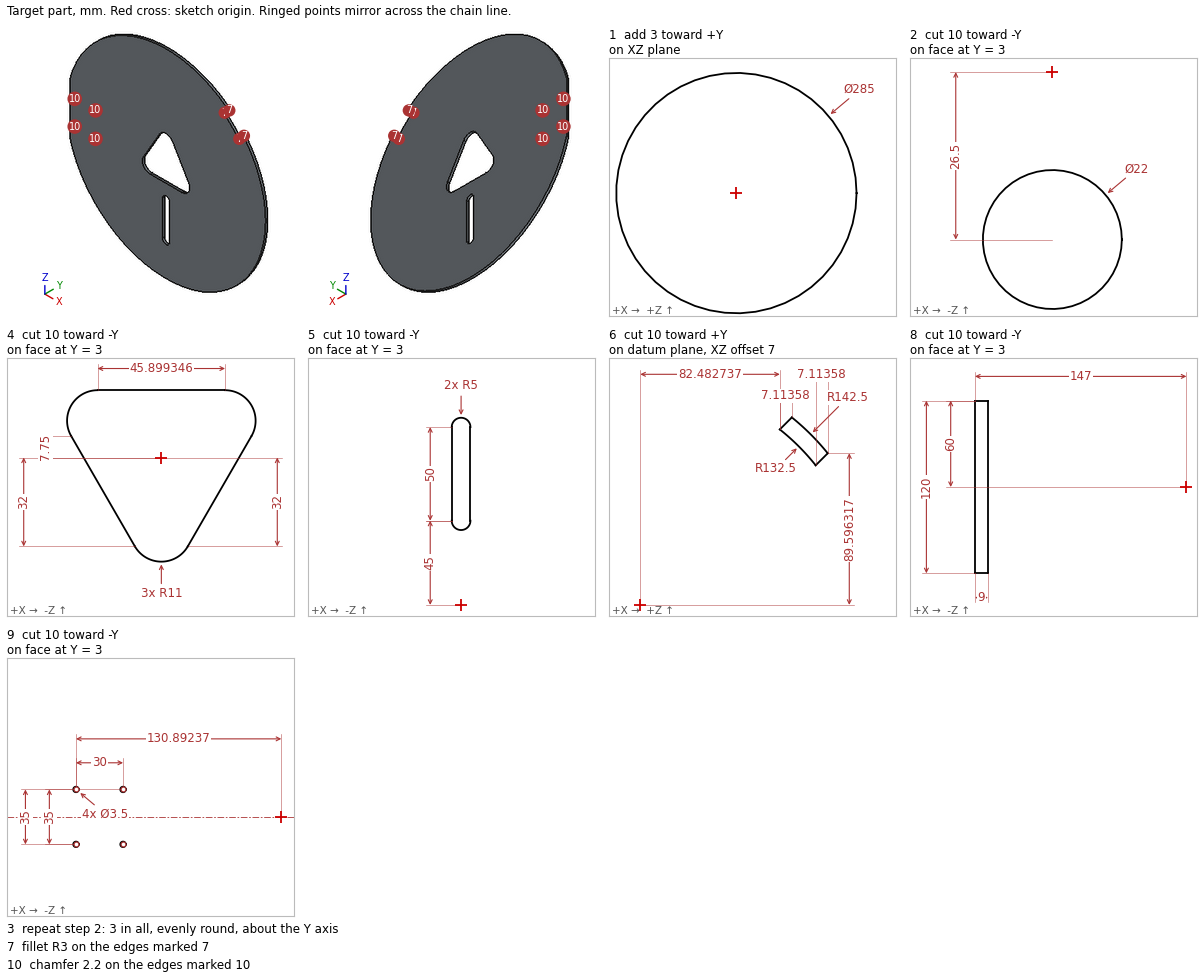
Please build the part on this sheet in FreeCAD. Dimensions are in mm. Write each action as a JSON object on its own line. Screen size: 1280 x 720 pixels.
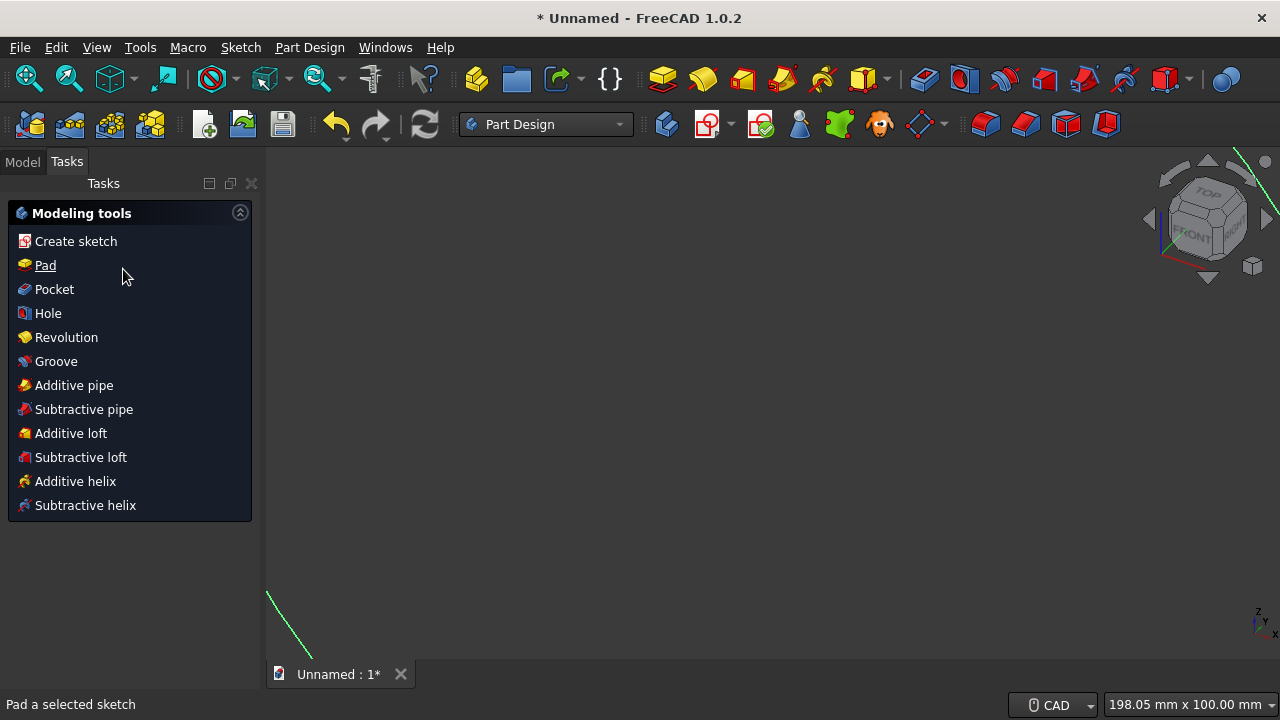
{"action": "left_click", "coordinate": [664, 80]}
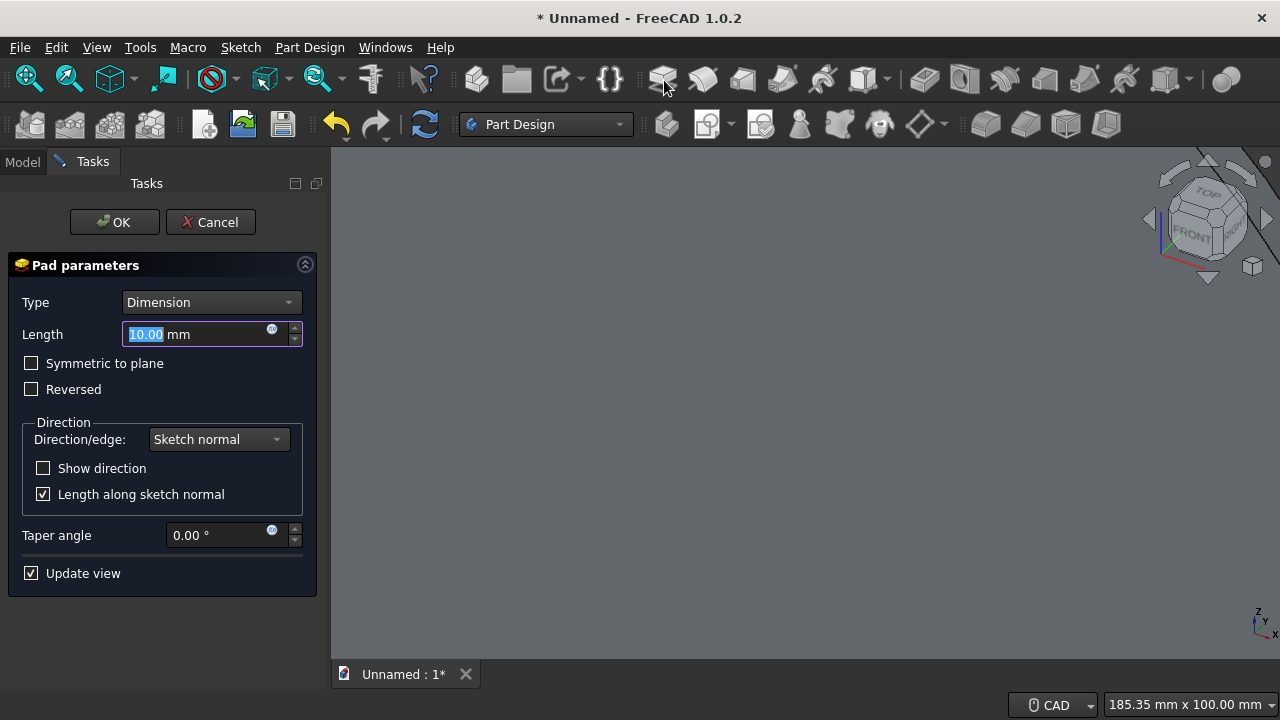
{"action": "type", "text": "3"}
{"action": "key", "text": "Tab"}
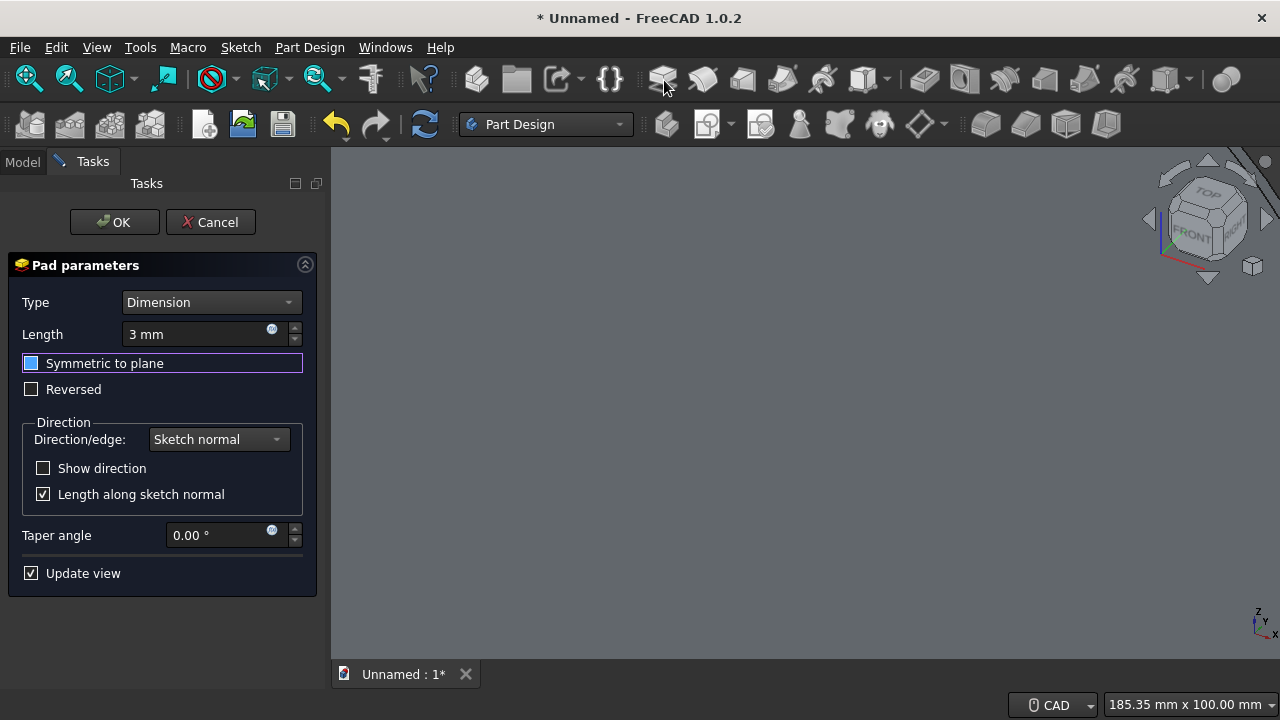
{"action": "left_click", "coordinate": [30, 389]}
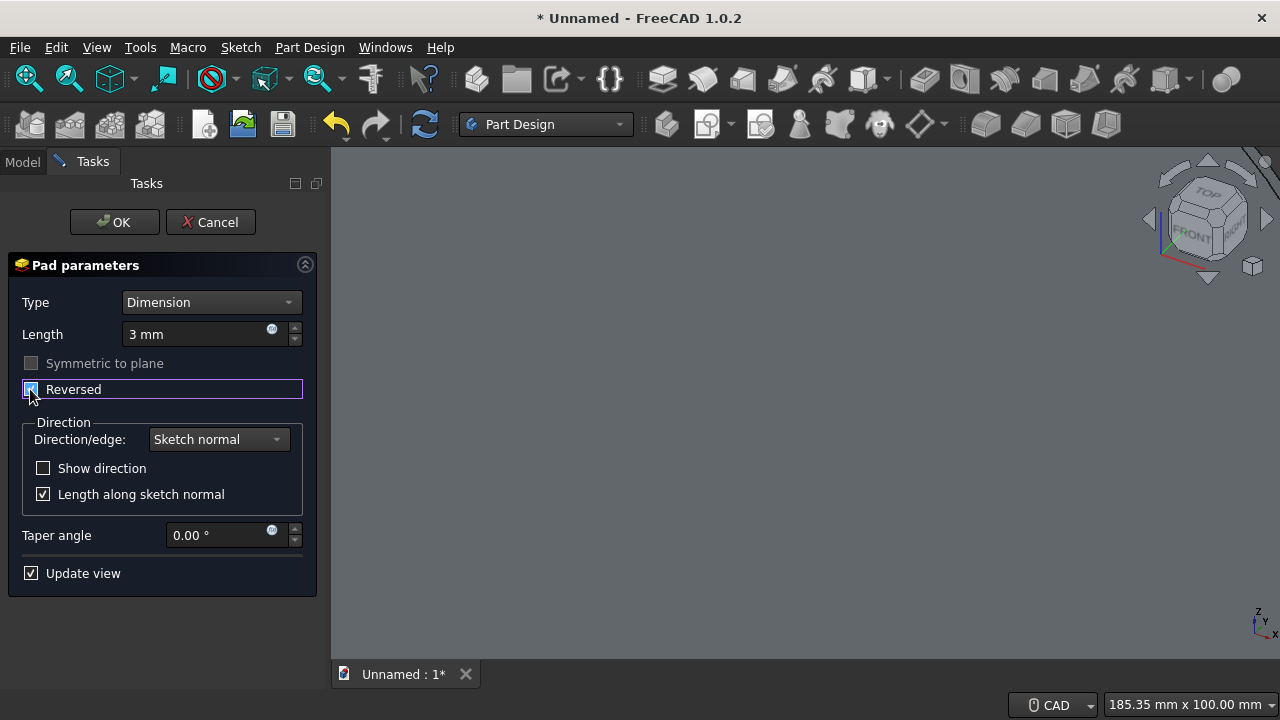
{"action": "left_click", "coordinate": [115, 222]}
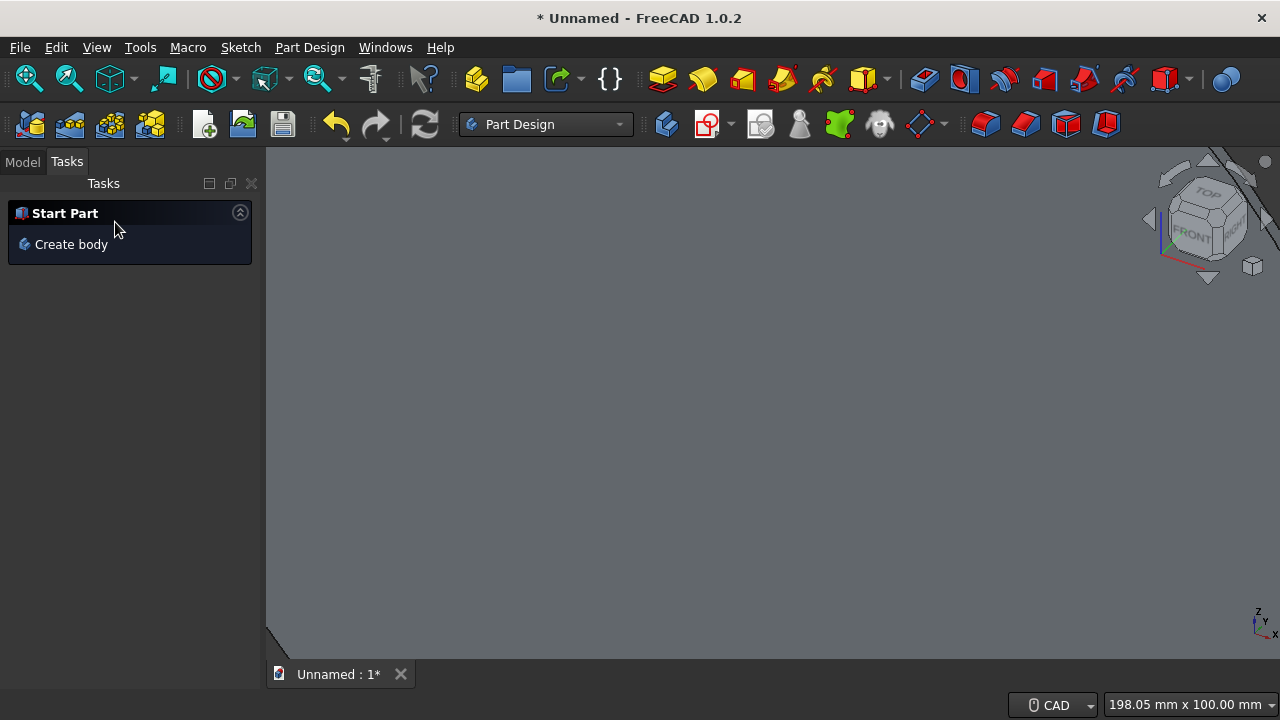
{"action": "left_click", "coordinate": [30, 80]}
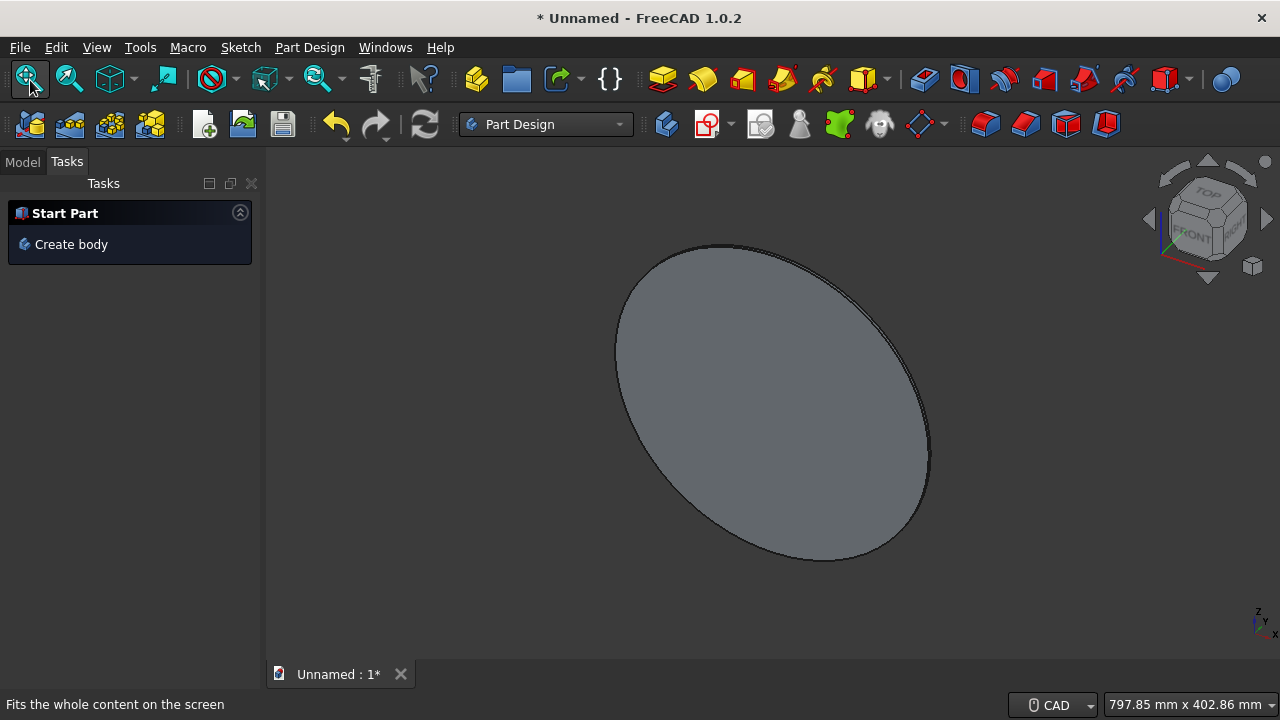
{"action": "key", "text": "4"}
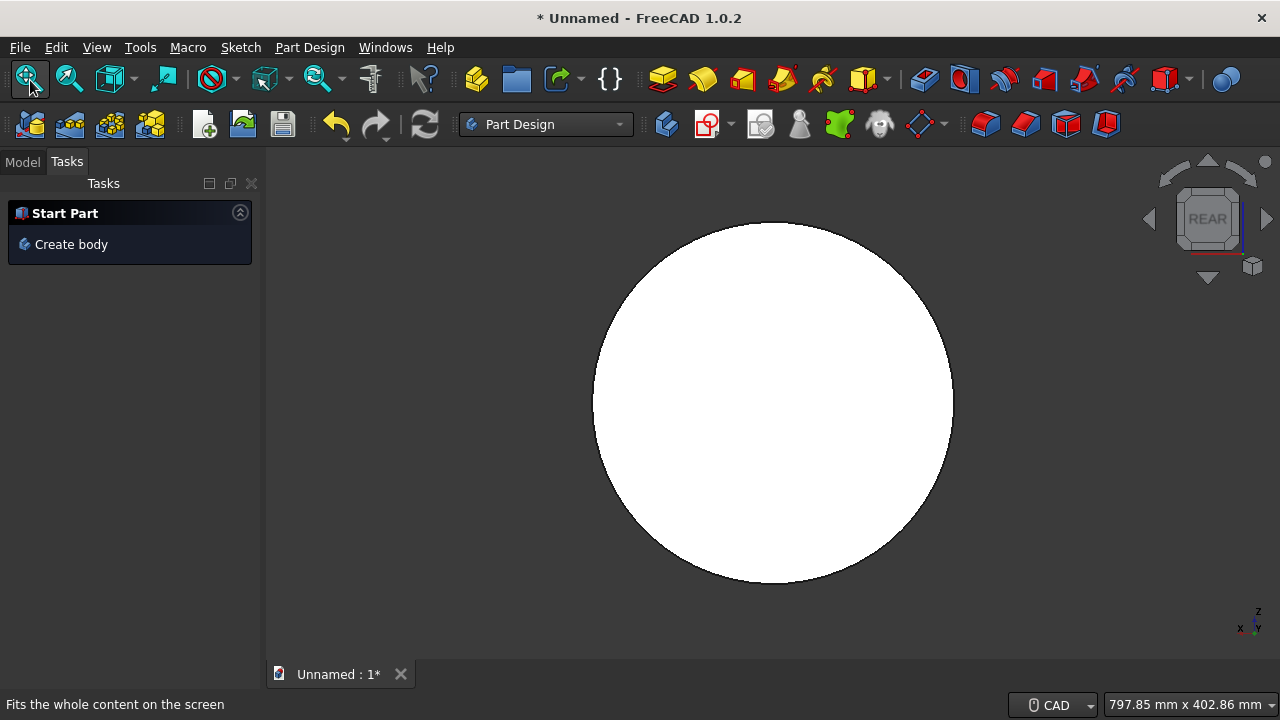
{"action": "left_click", "coordinate": [773, 402]}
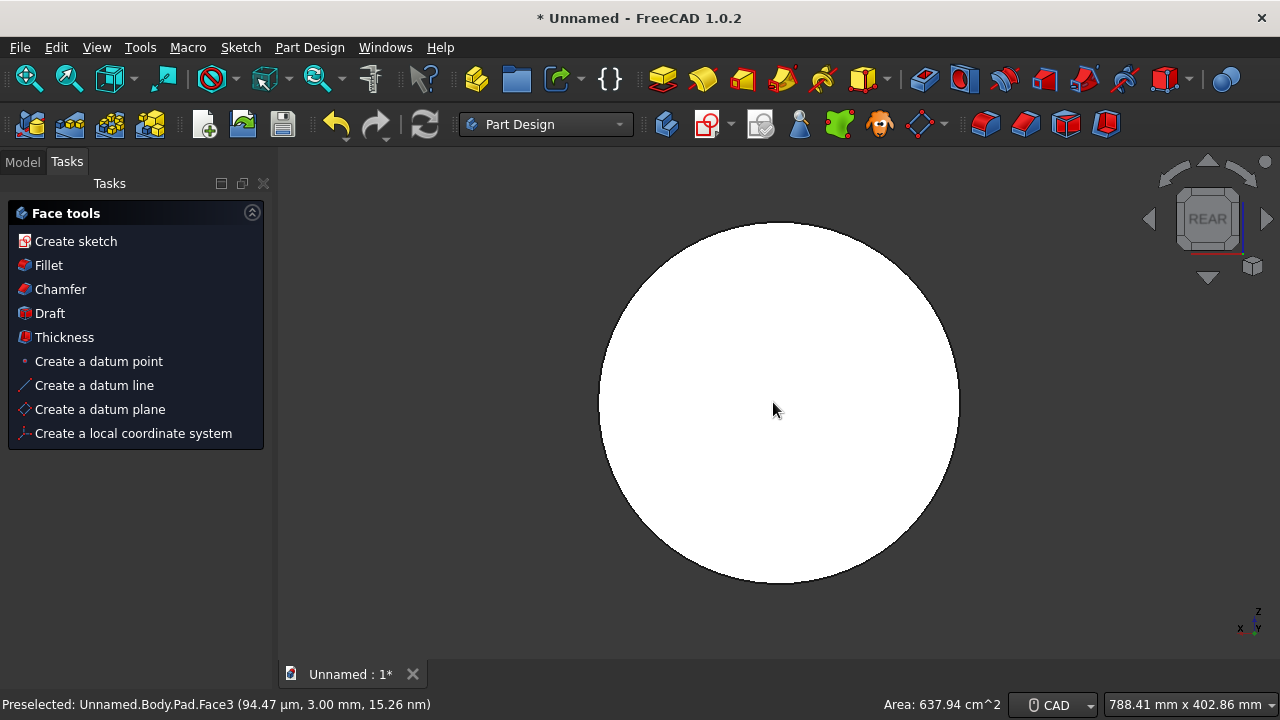
{"action": "left_click", "coordinate": [708, 124]}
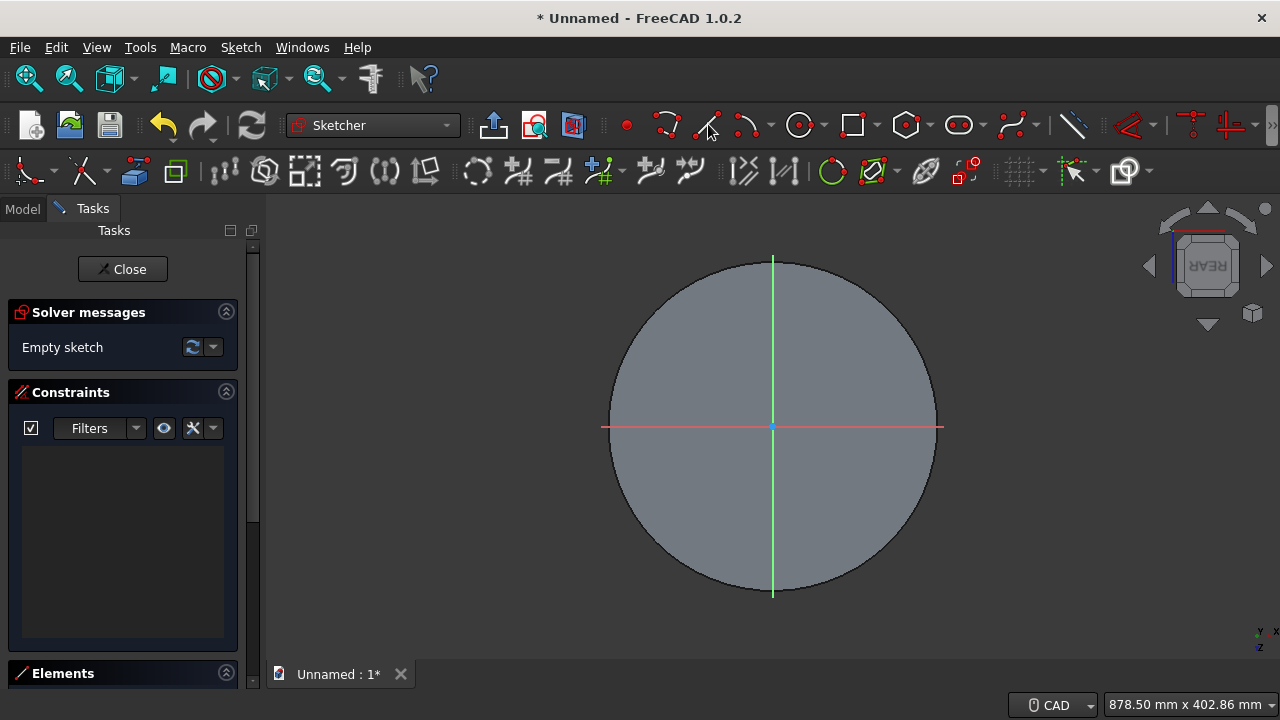
{"action": "scroll", "coordinate": [786, 452], "scroll_direction": "up", "scroll_amount": 9}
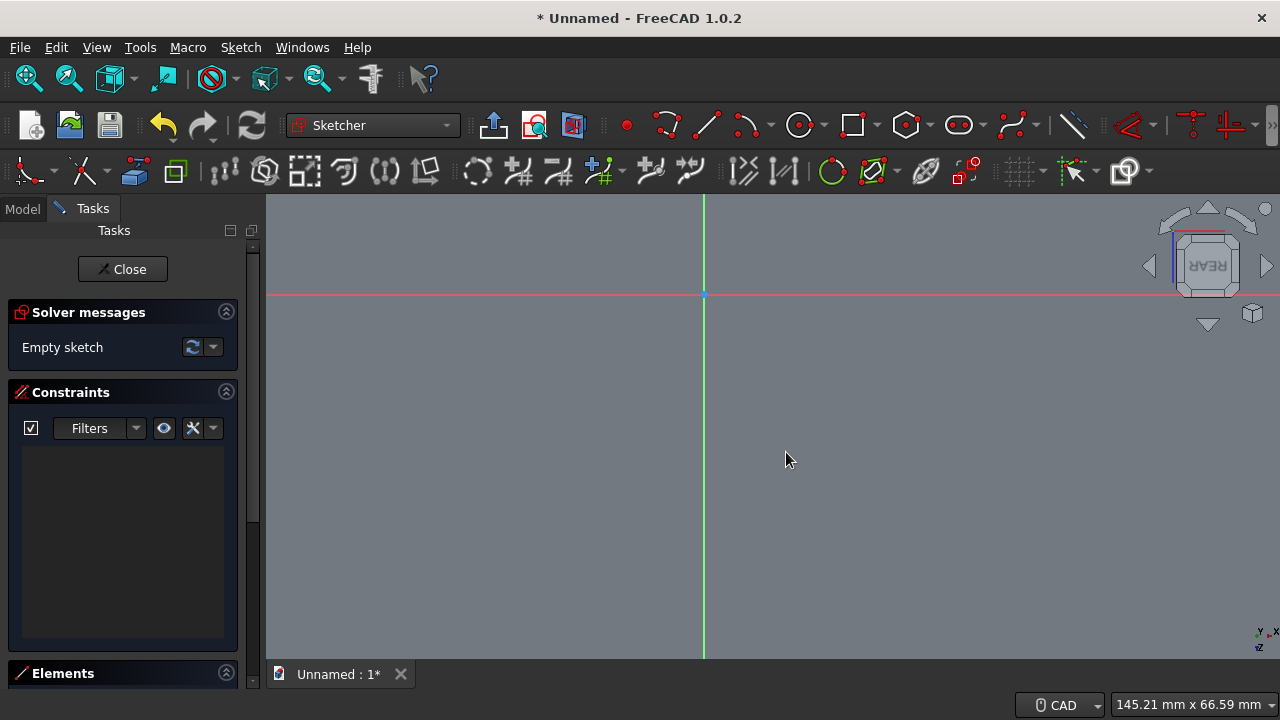
{"action": "left_click", "coordinate": [800, 126]}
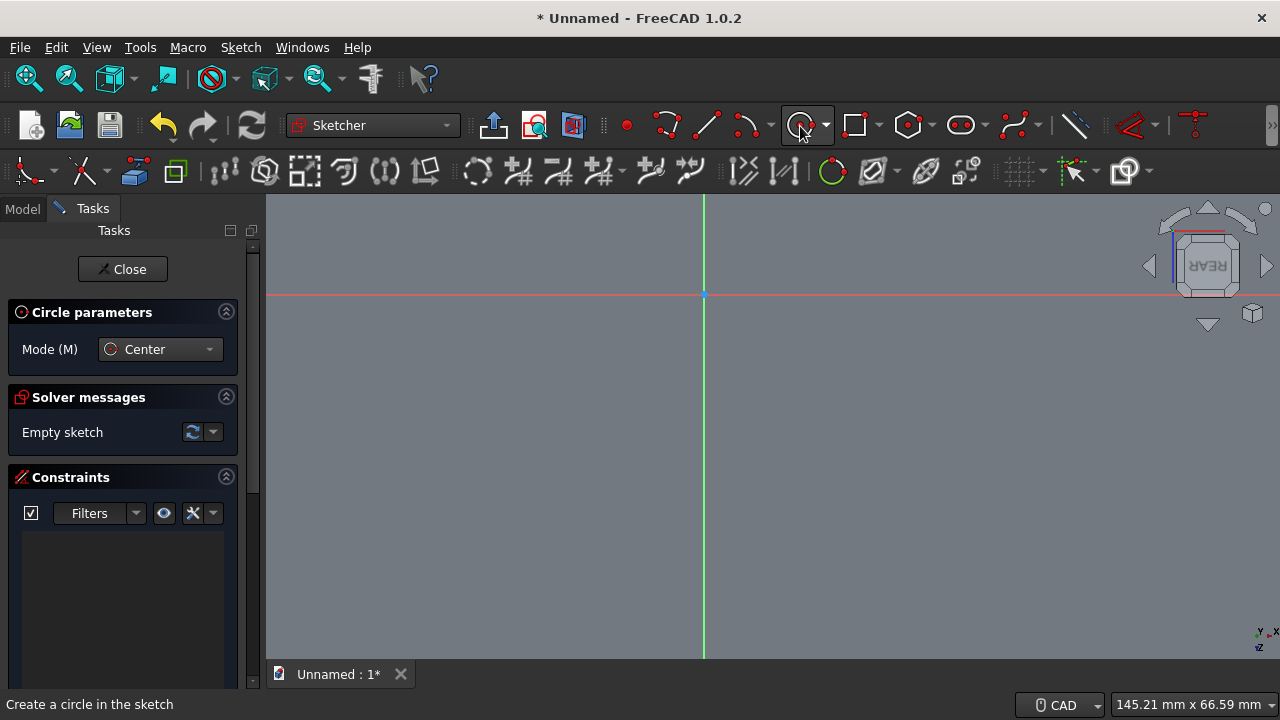
{"action": "left_click", "coordinate": [704, 480]}
{"action": "left_click", "coordinate": [758, 426]}
{"action": "key", "text": "Escape"}